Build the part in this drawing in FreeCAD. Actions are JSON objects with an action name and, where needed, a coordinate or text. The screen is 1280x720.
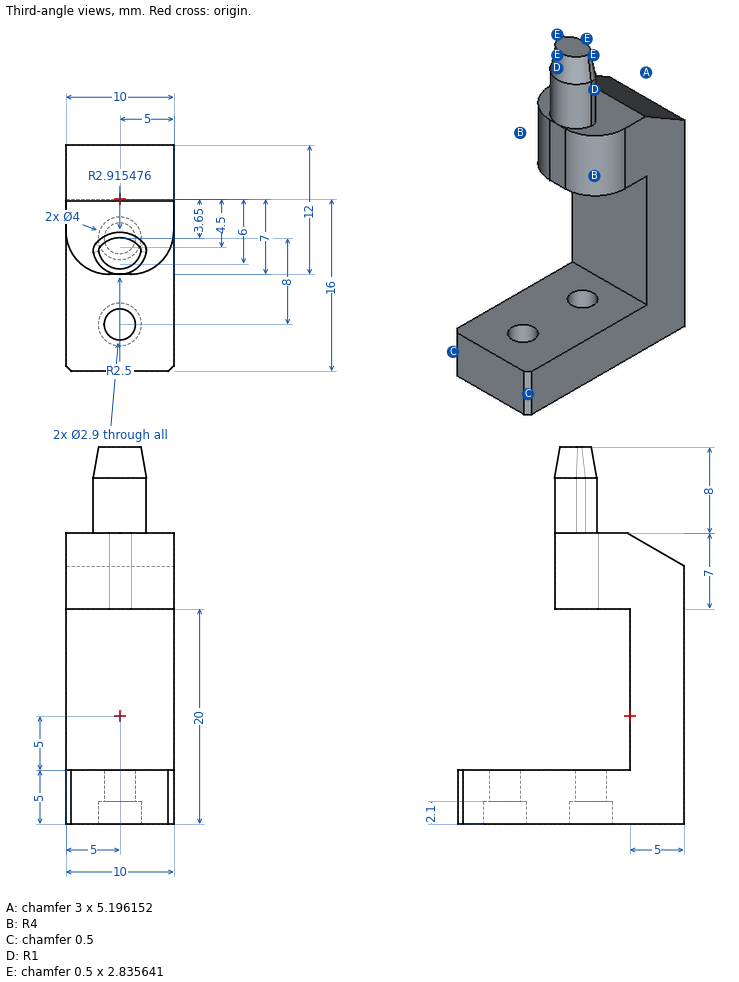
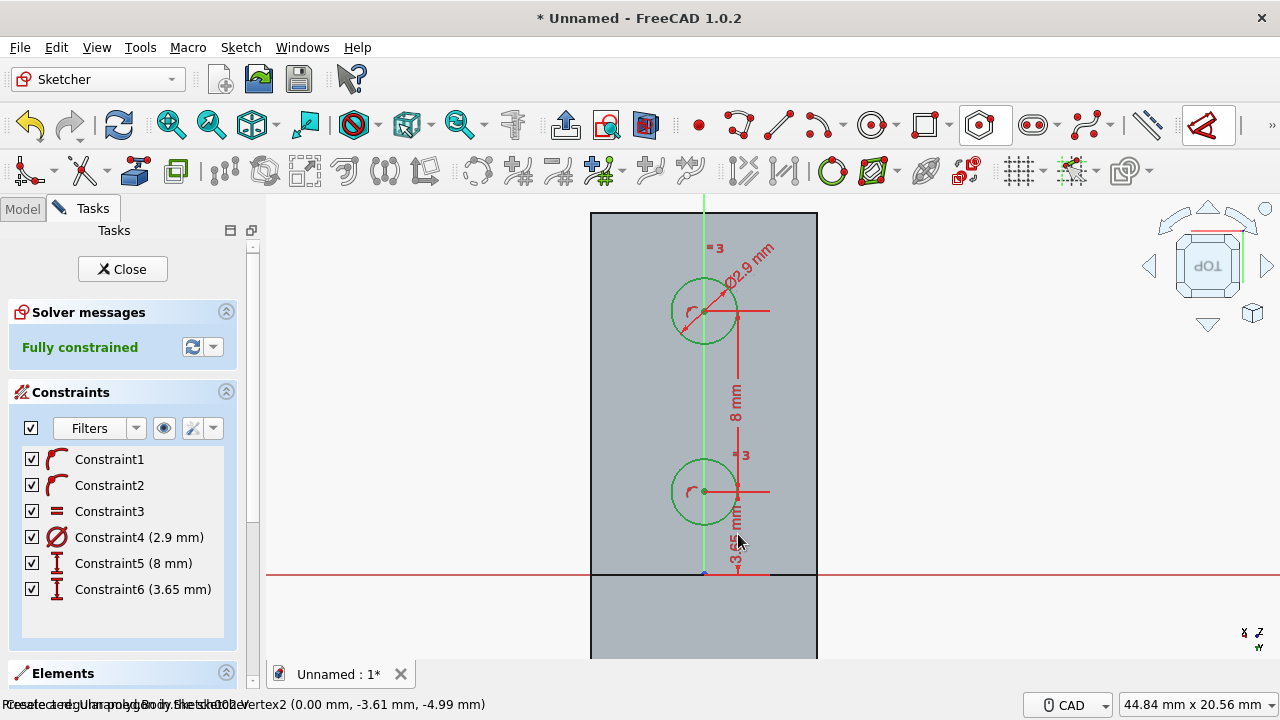
{"action": "left_click", "coordinate": [123, 269]}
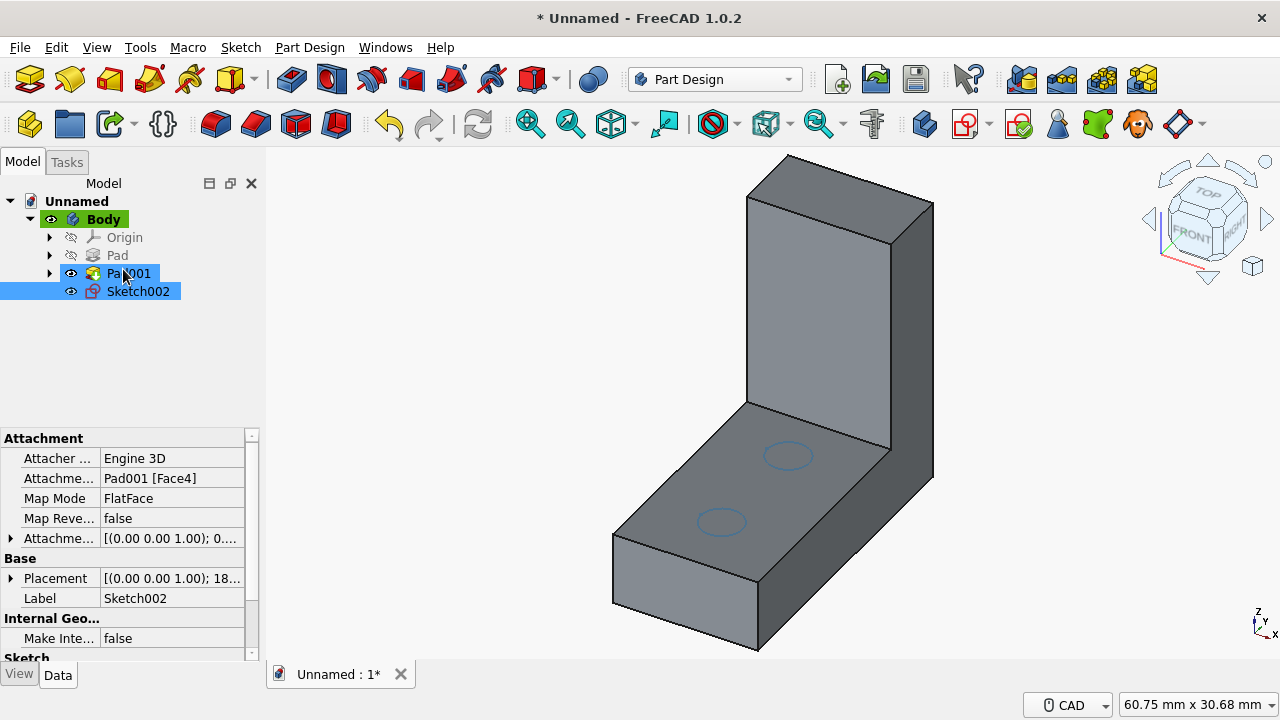
{"action": "left_click", "coordinate": [332, 80]}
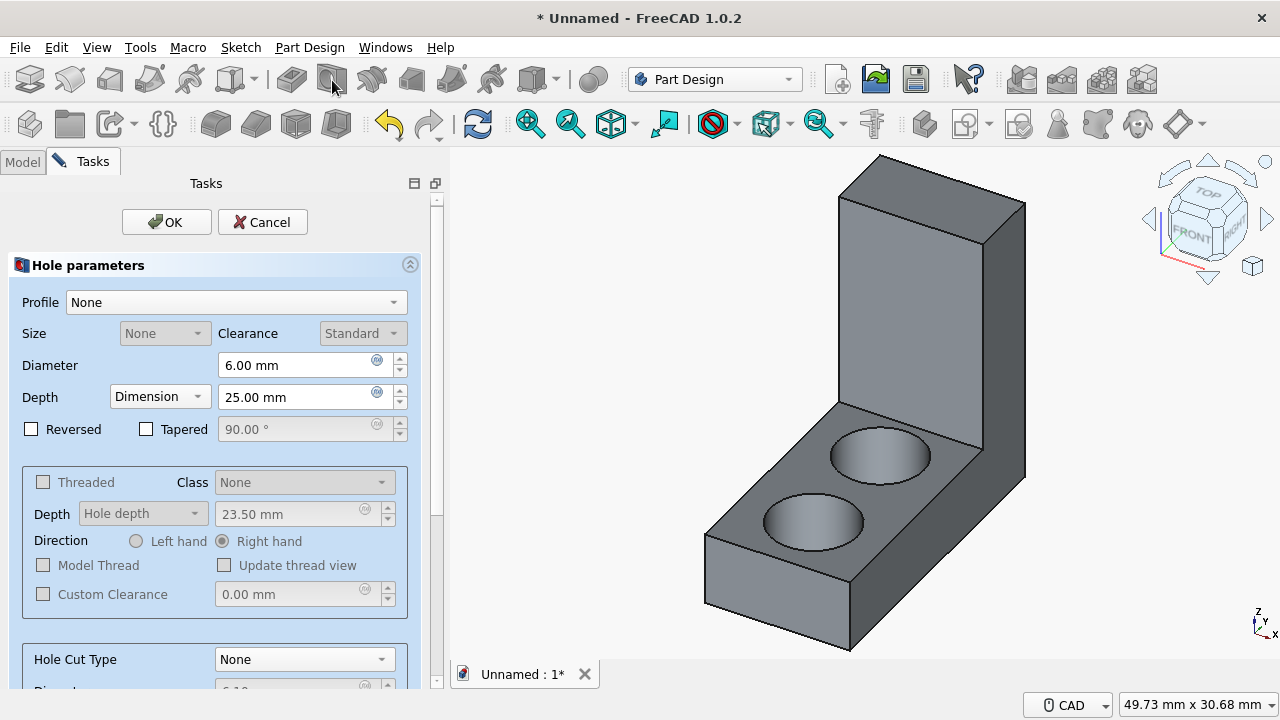
{"action": "triple_click", "coordinate": [305, 365]}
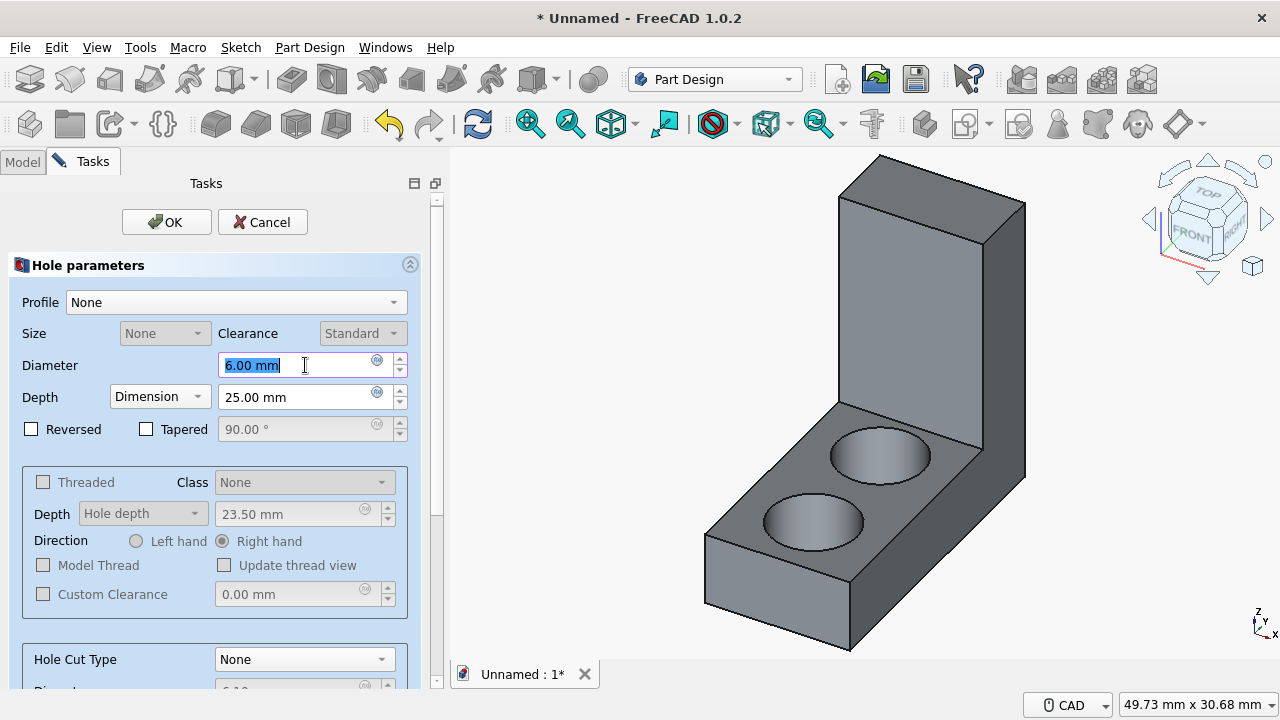
{"action": "type", "text": "2.9"}
{"action": "key", "text": "Tab"}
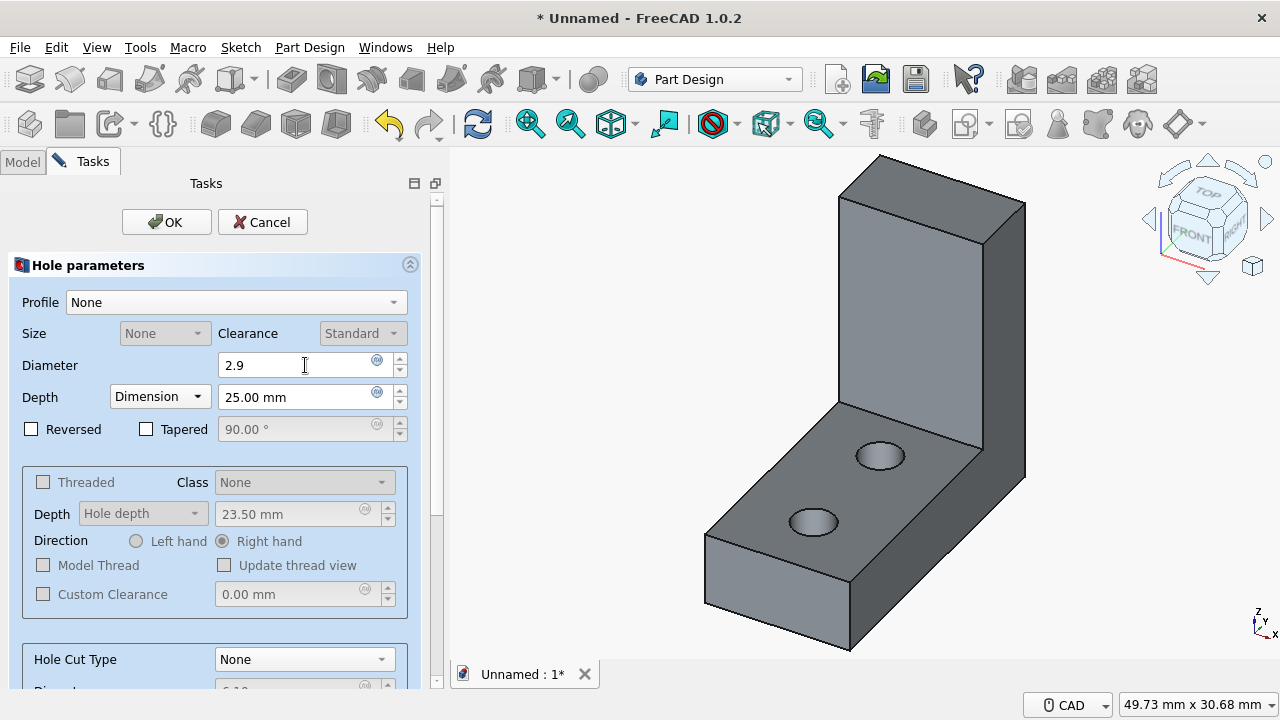
{"action": "left_click", "coordinate": [161, 396]}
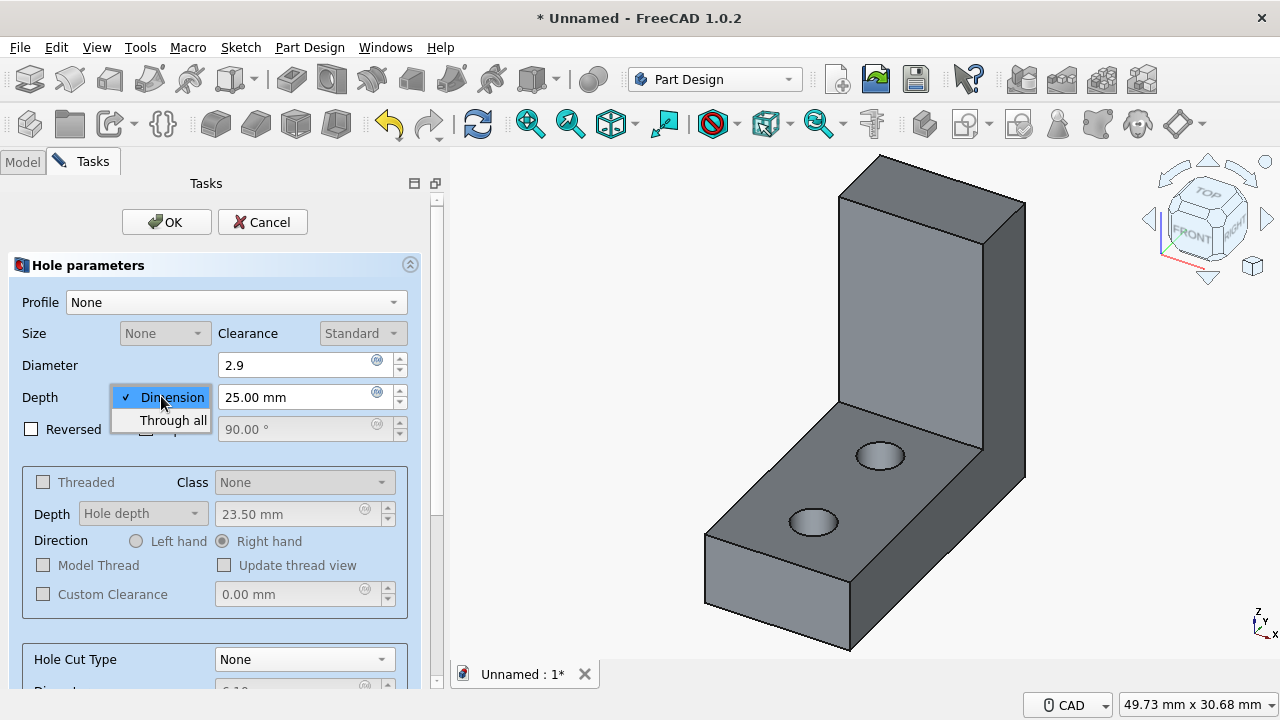
{"action": "left_click", "coordinate": [160, 420]}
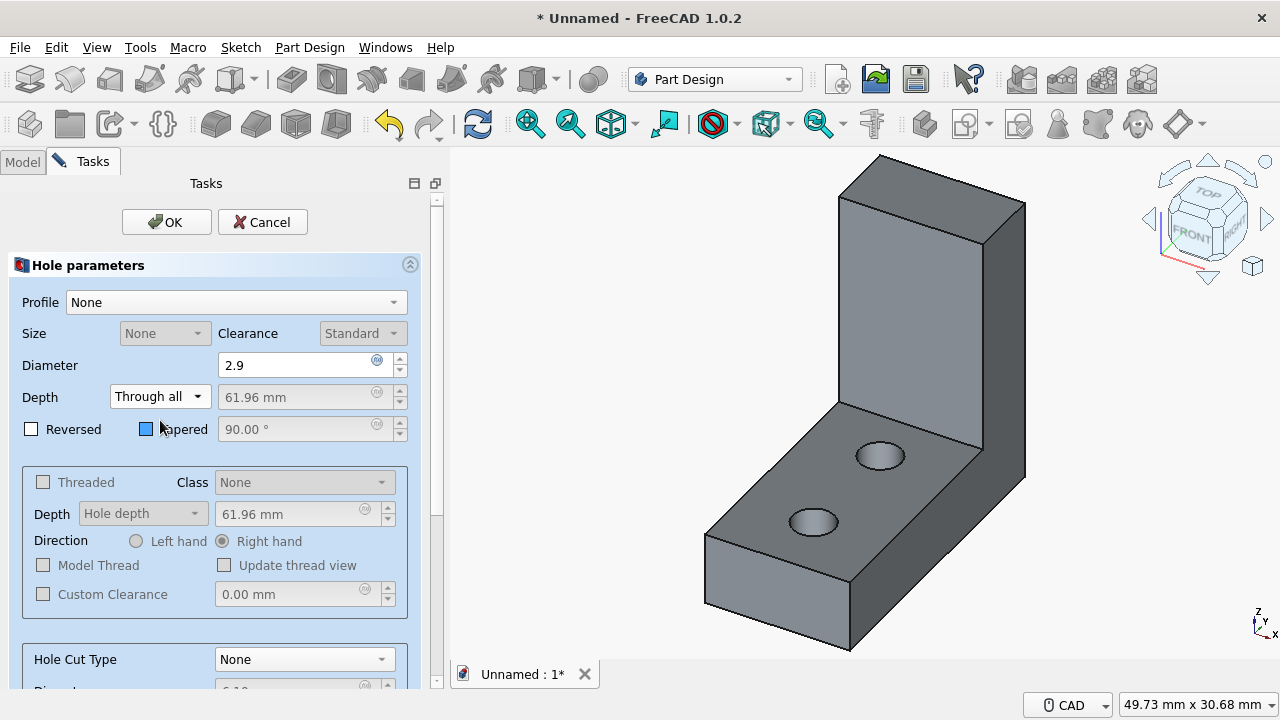
{"action": "left_click", "coordinate": [167, 222]}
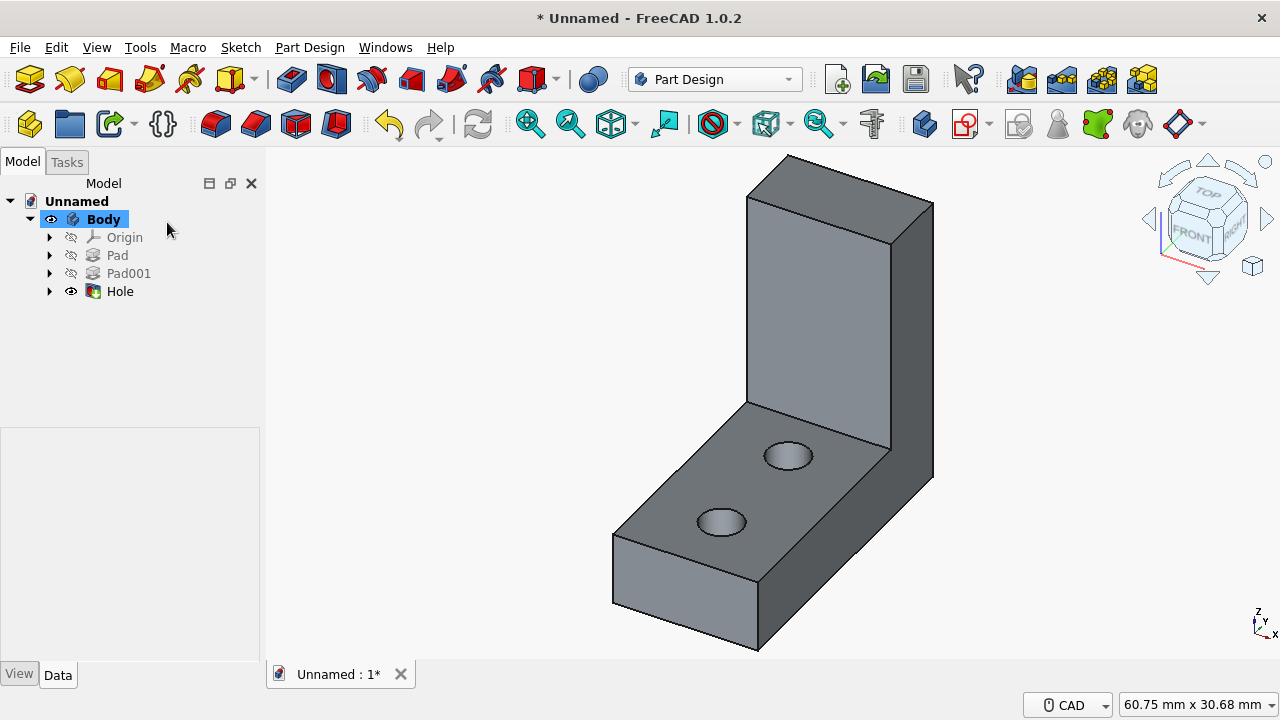
{"action": "left_click", "coordinate": [860, 206]}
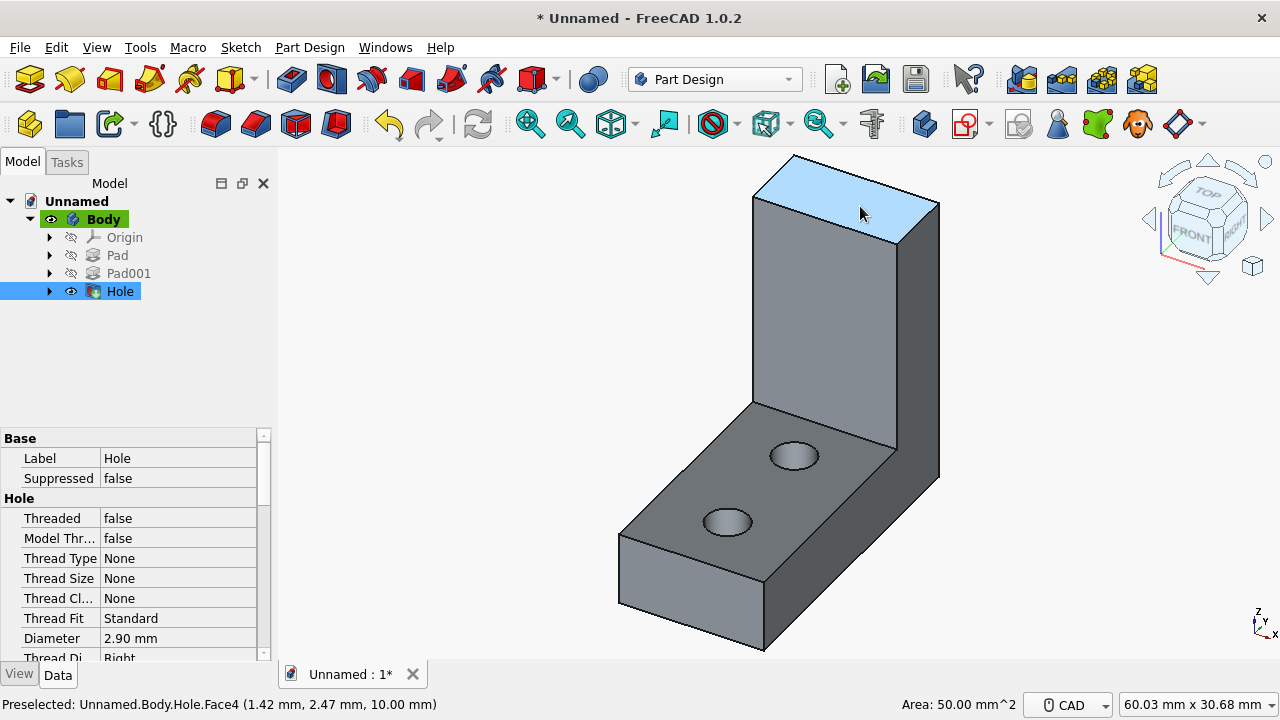
{"action": "left_click", "coordinate": [966, 124]}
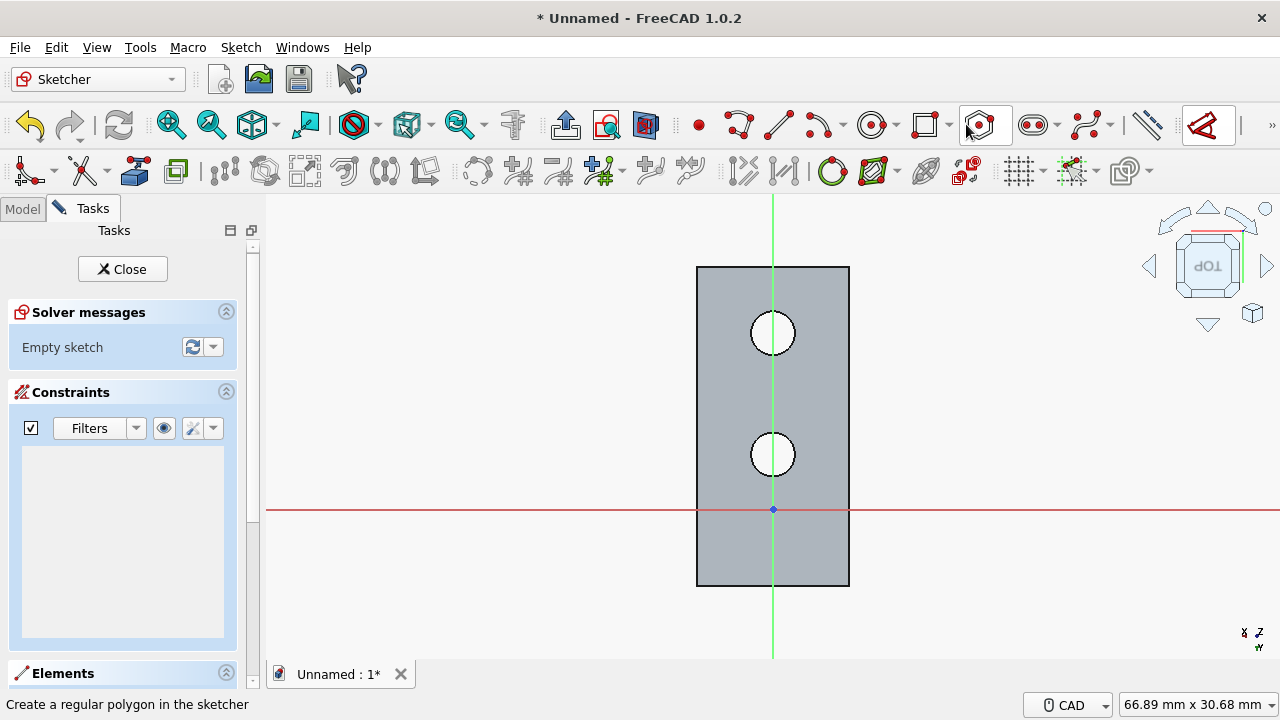
{"action": "scroll", "coordinate": [912, 631], "scroll_direction": "up", "scroll_amount": 2}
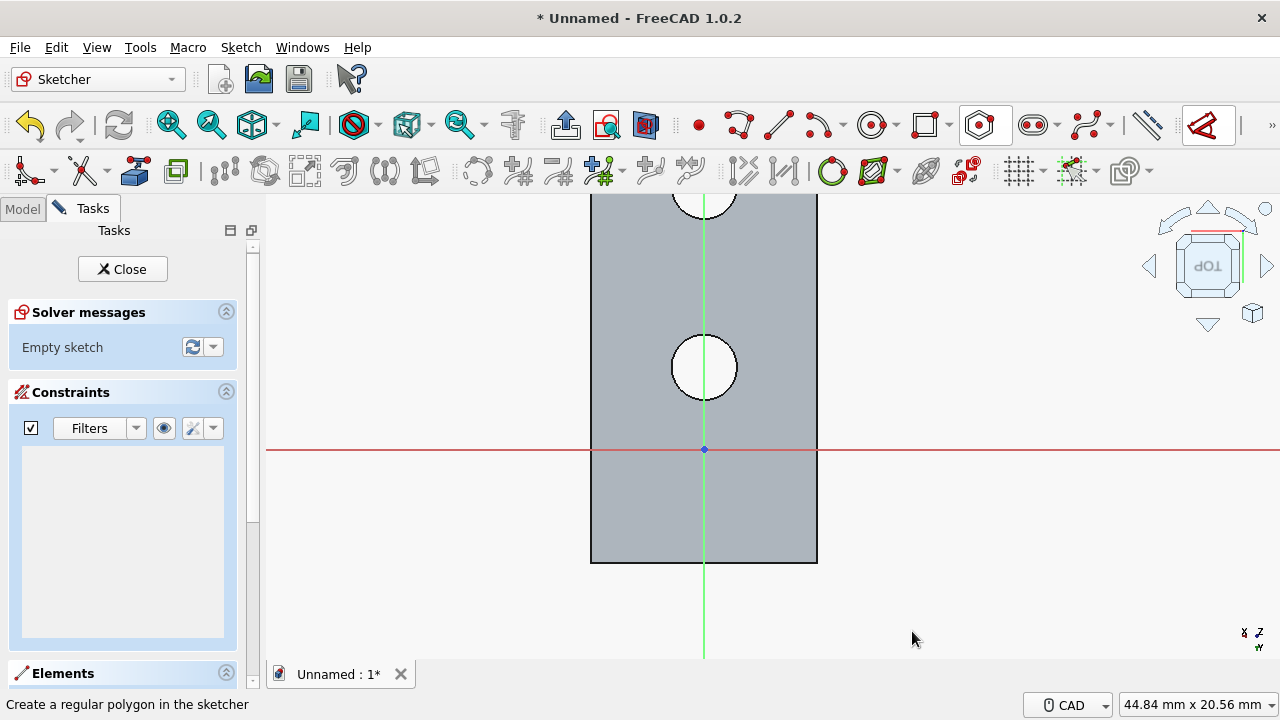
{"action": "left_click", "coordinate": [926, 126]}